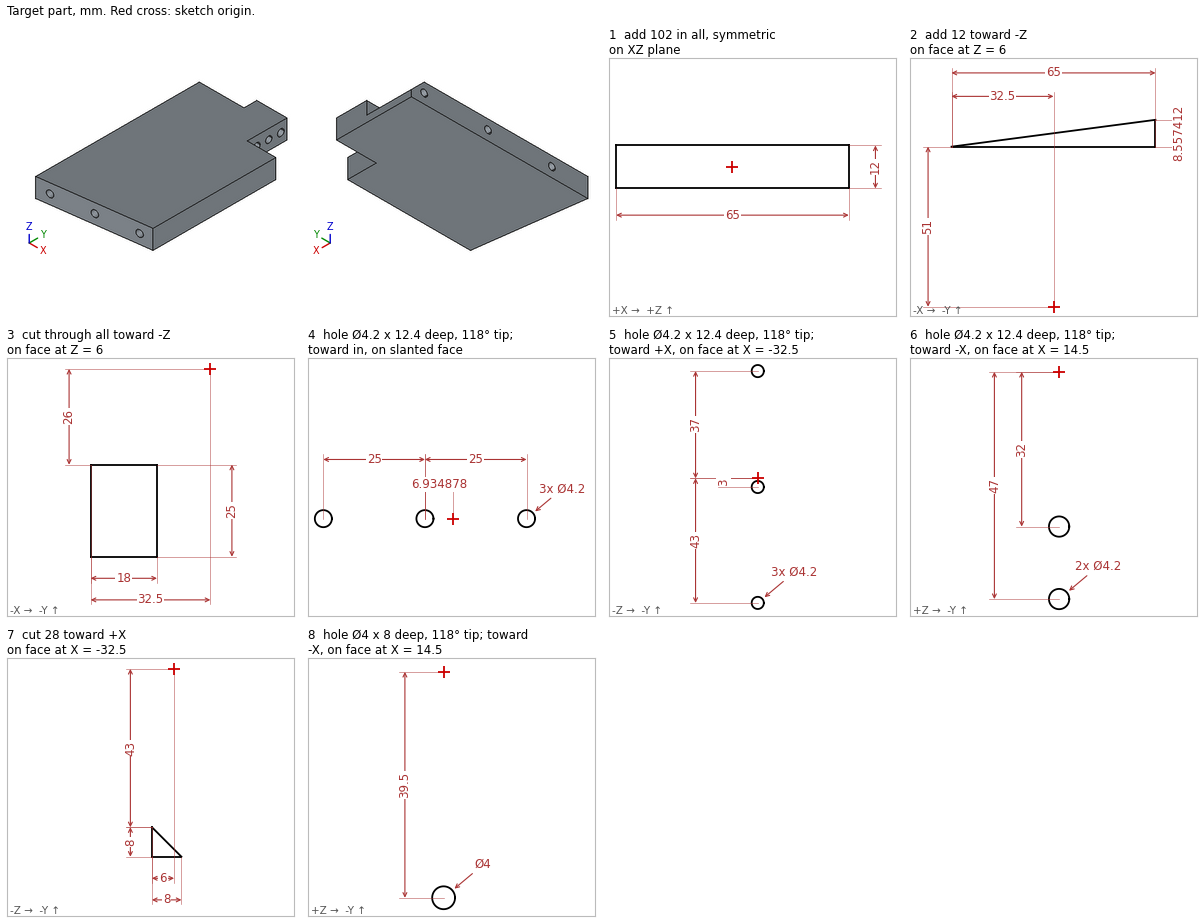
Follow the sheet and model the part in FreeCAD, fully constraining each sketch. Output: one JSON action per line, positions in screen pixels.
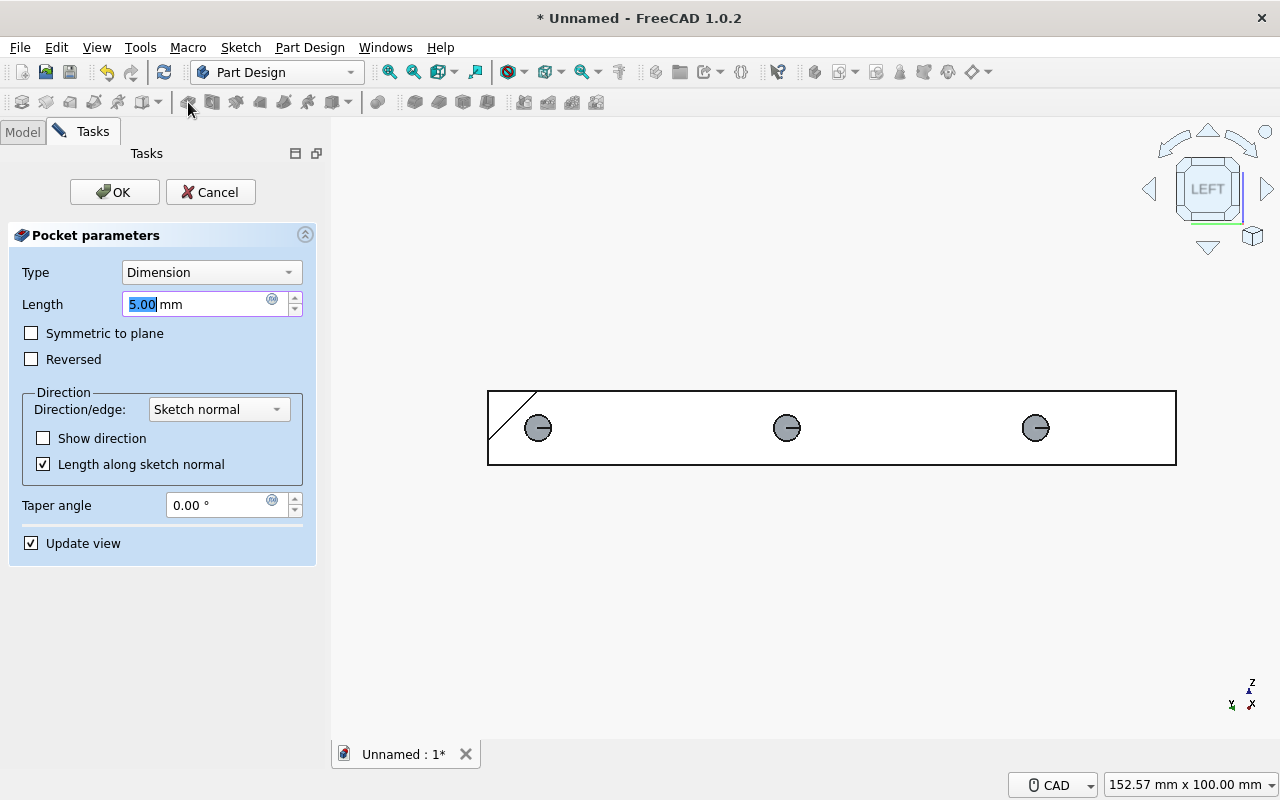
{"action": "type", "text": "28"}
{"action": "key", "text": "Tab"}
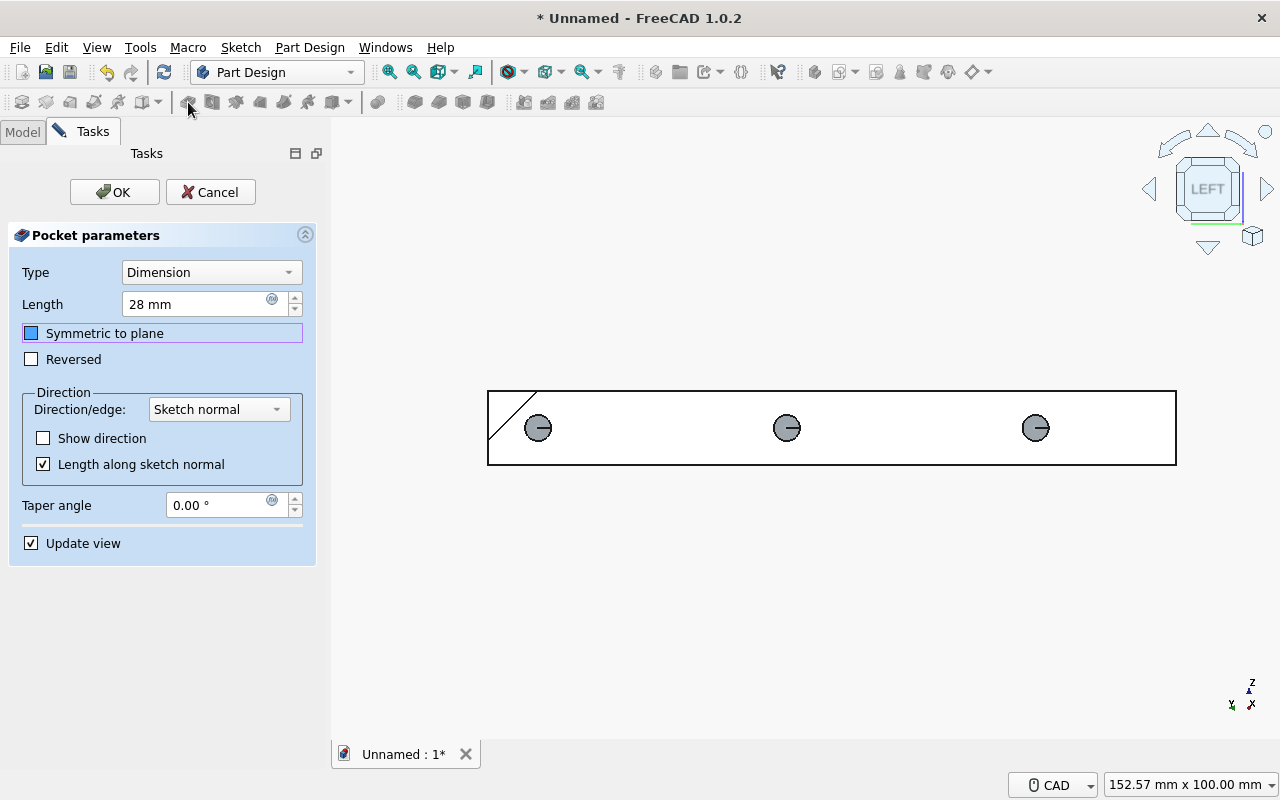
{"action": "left_click", "coordinate": [115, 192]}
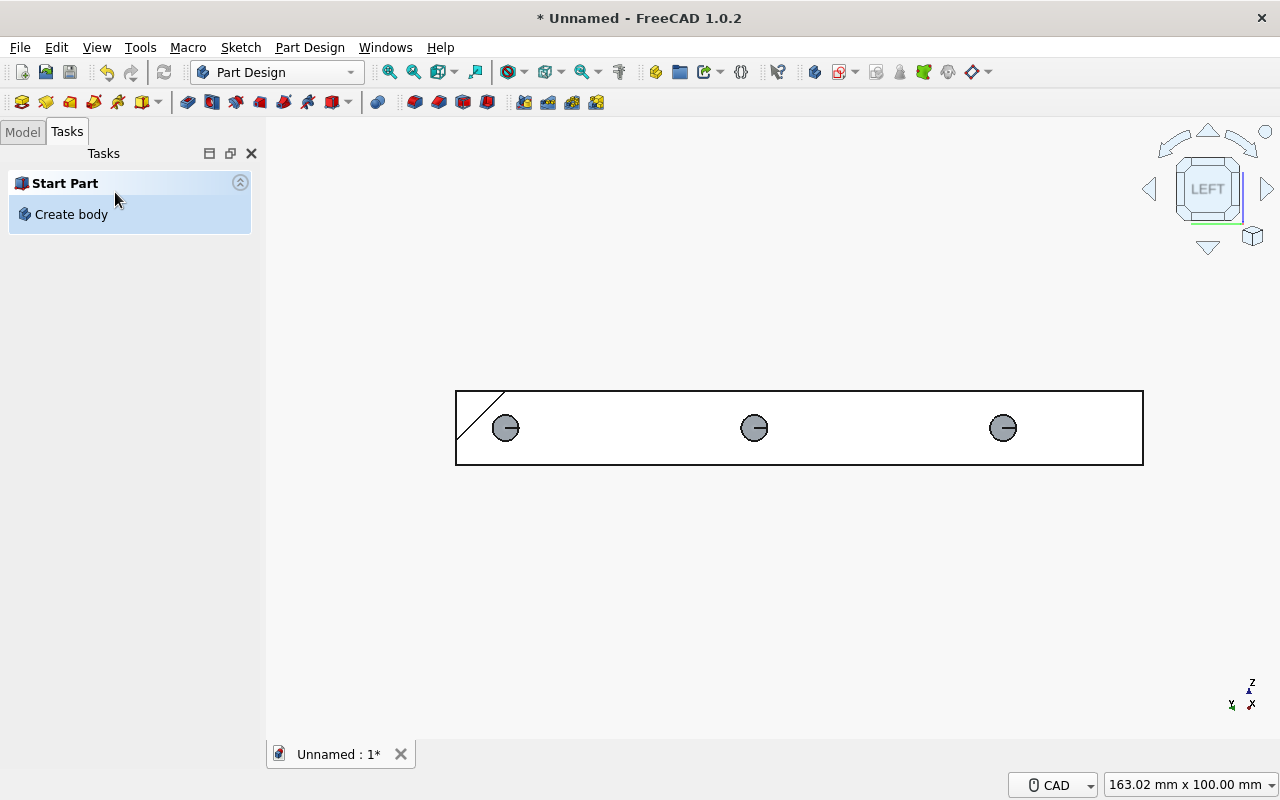
{"action": "key", "text": "0"}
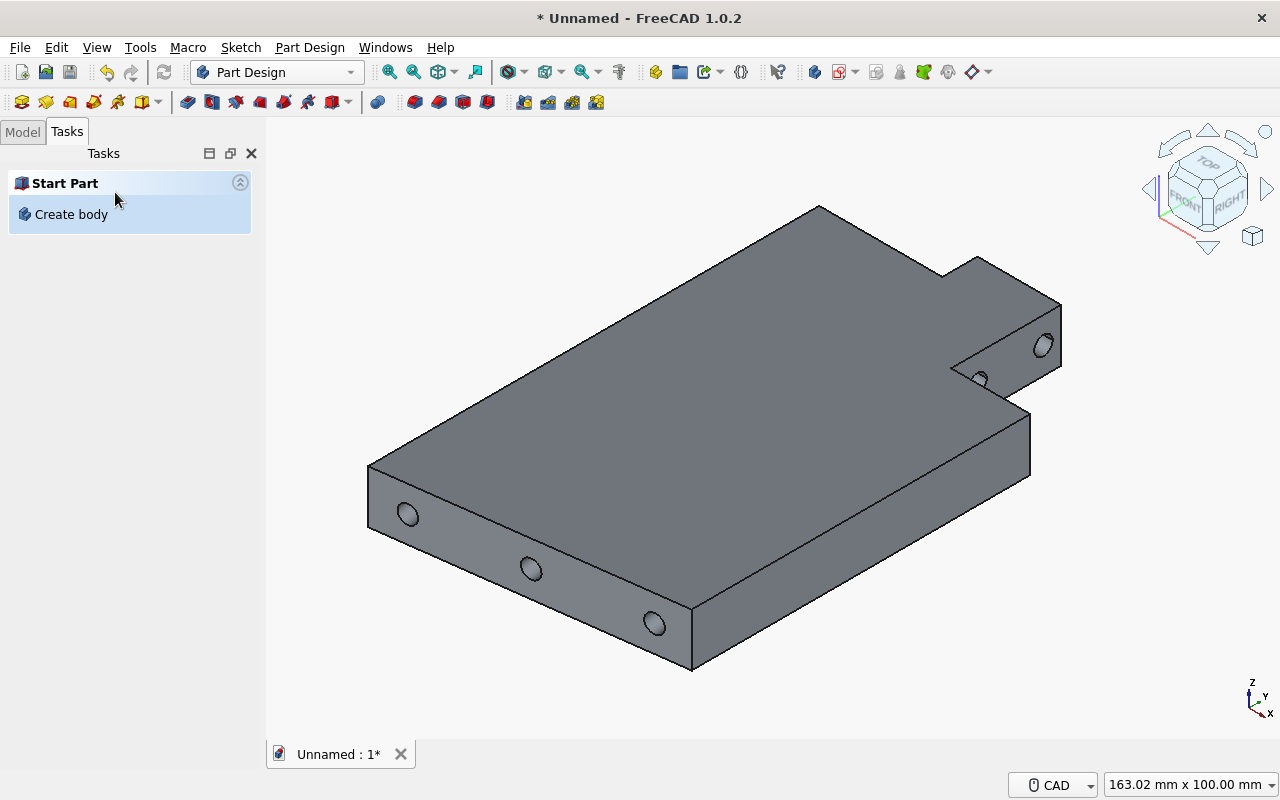
{"action": "left_click", "coordinate": [1006, 366]}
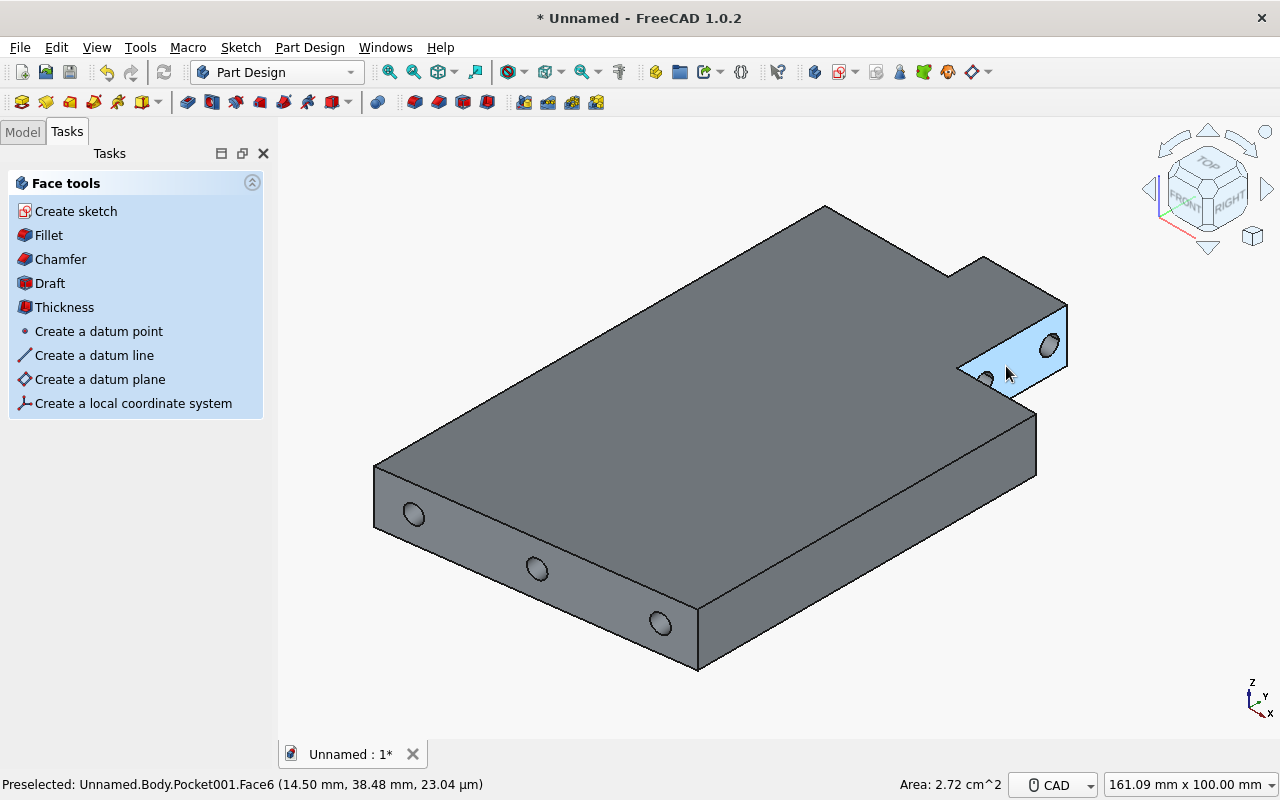
{"action": "left_click", "coordinate": [840, 72]}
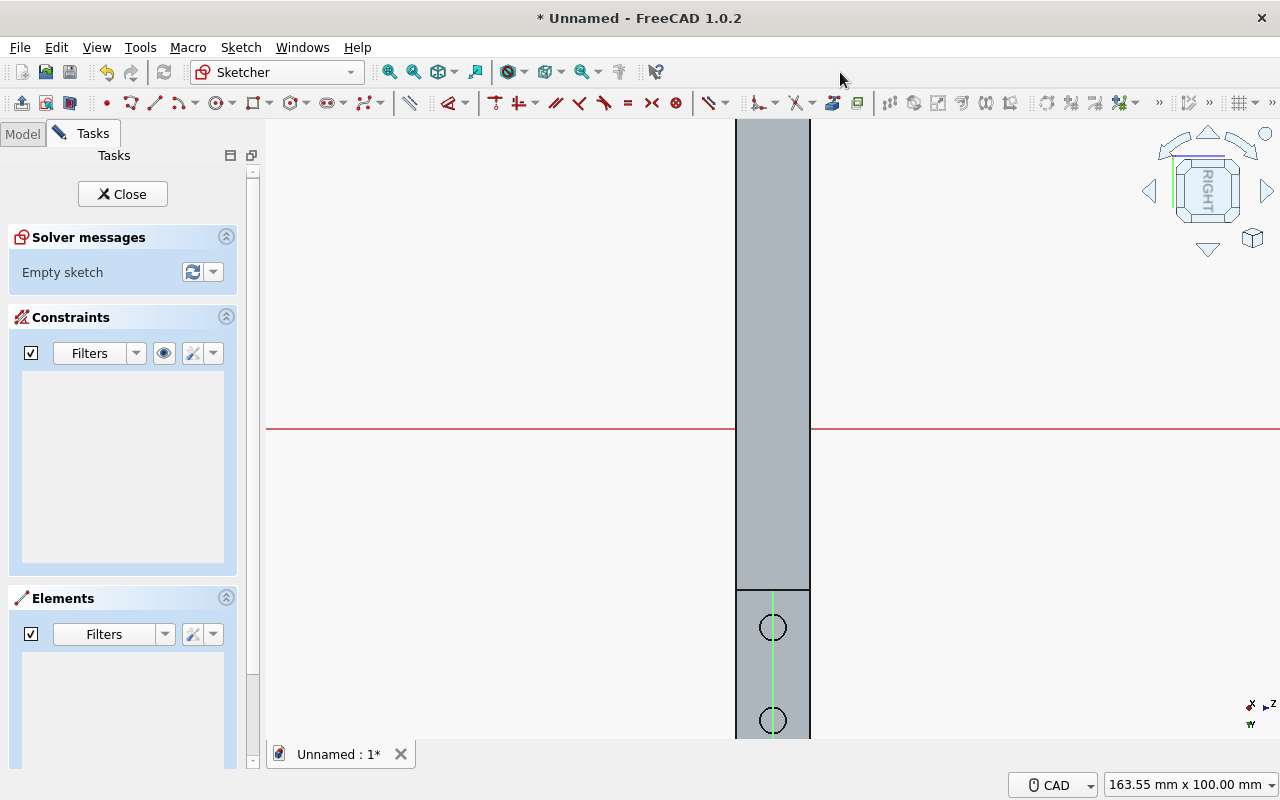
{"action": "scroll", "coordinate": [777, 690], "scroll_direction": "up", "scroll_amount": 14}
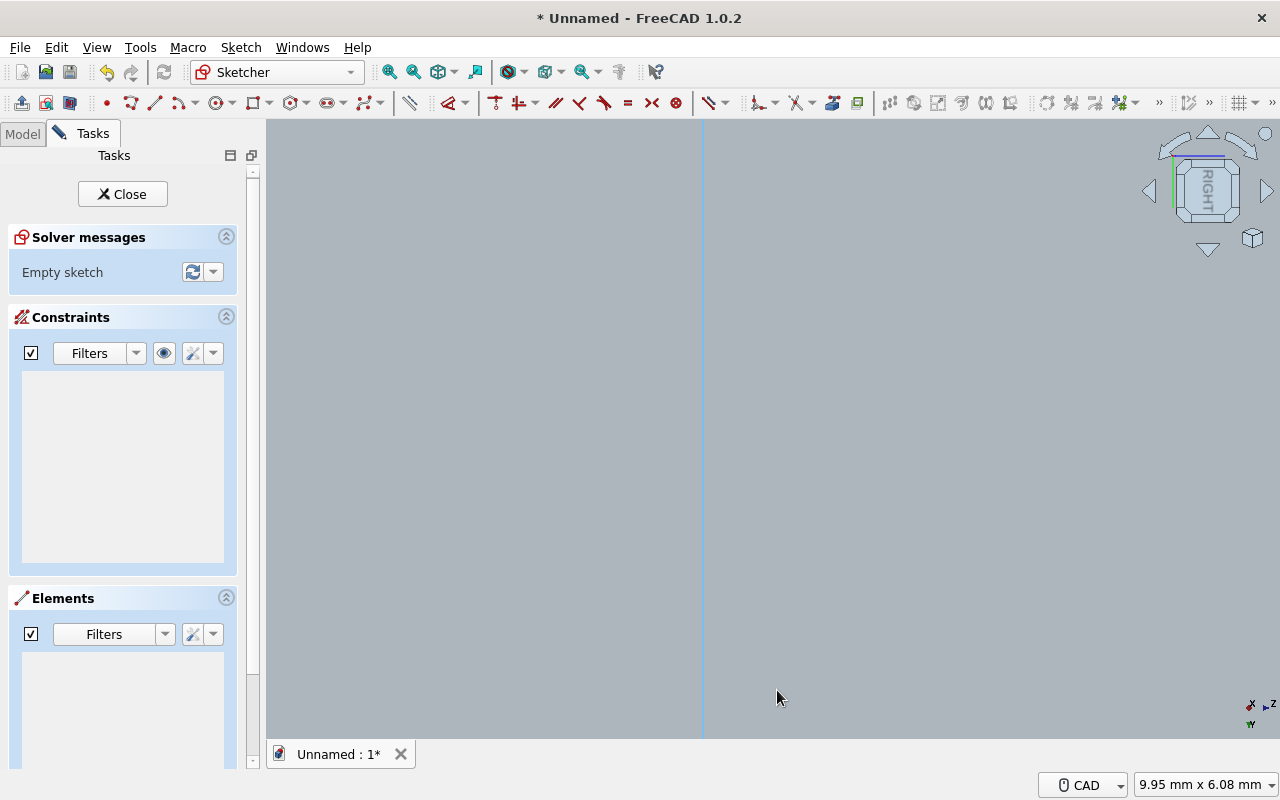
{"action": "key", "text": "g c"}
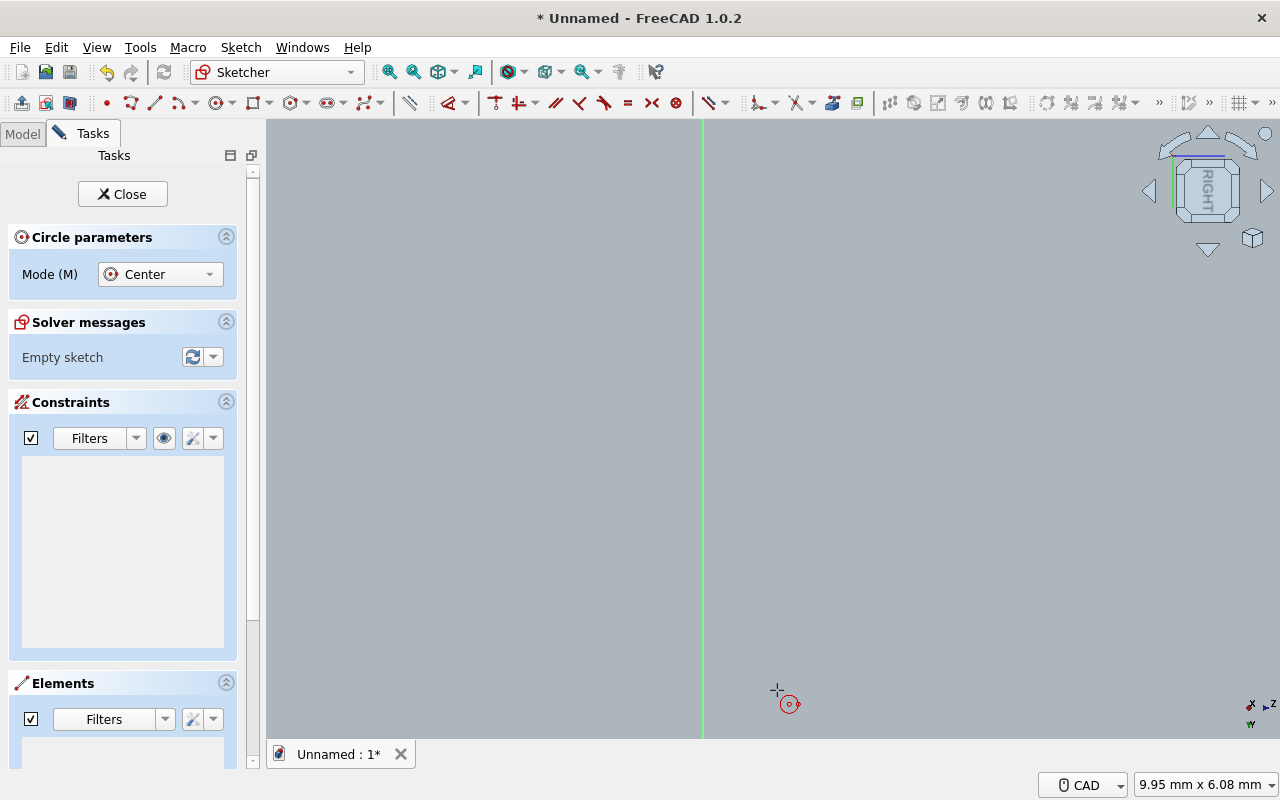
{"action": "left_click", "coordinate": [703, 411]}
{"action": "mouse_move", "coordinate": [848, 267]}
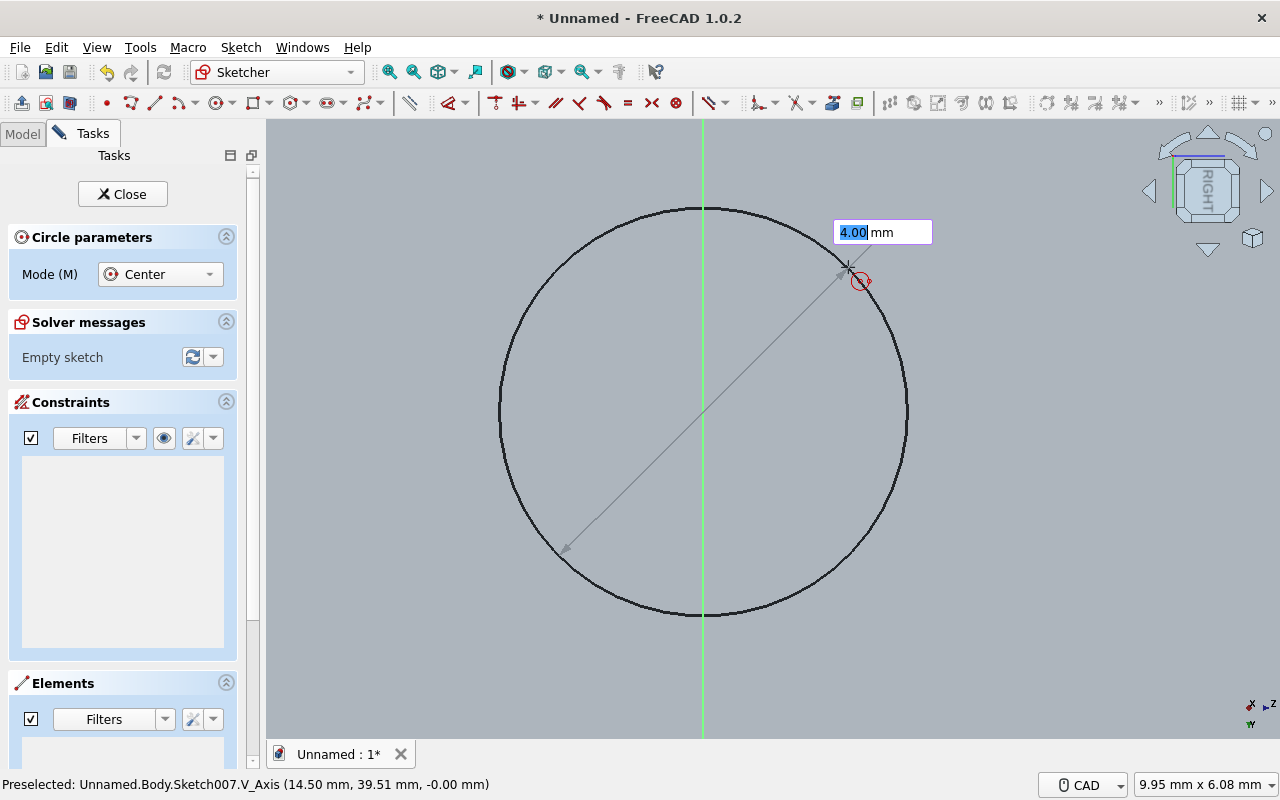
{"action": "type", "text": "4"}
{"action": "key", "text": "Return"}
{"action": "key", "text": "Escape"}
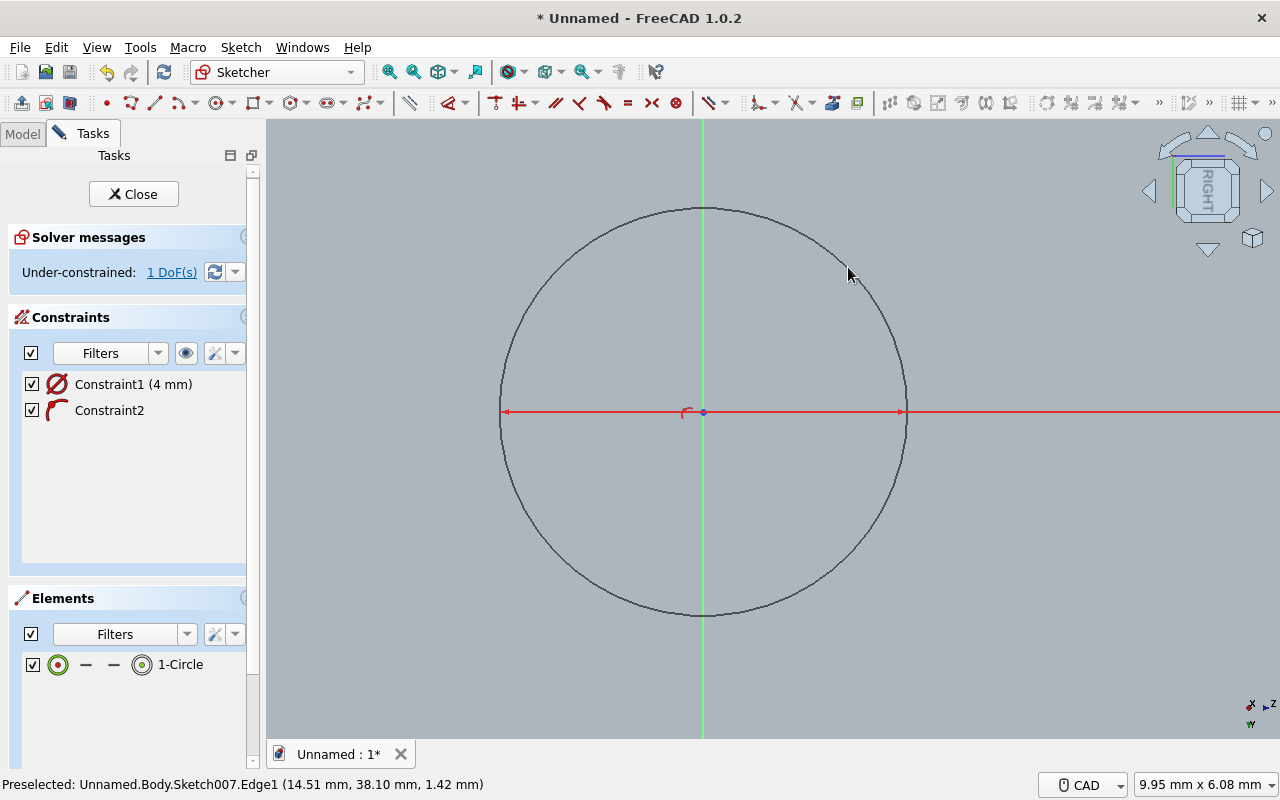
{"action": "key", "text": "d"}